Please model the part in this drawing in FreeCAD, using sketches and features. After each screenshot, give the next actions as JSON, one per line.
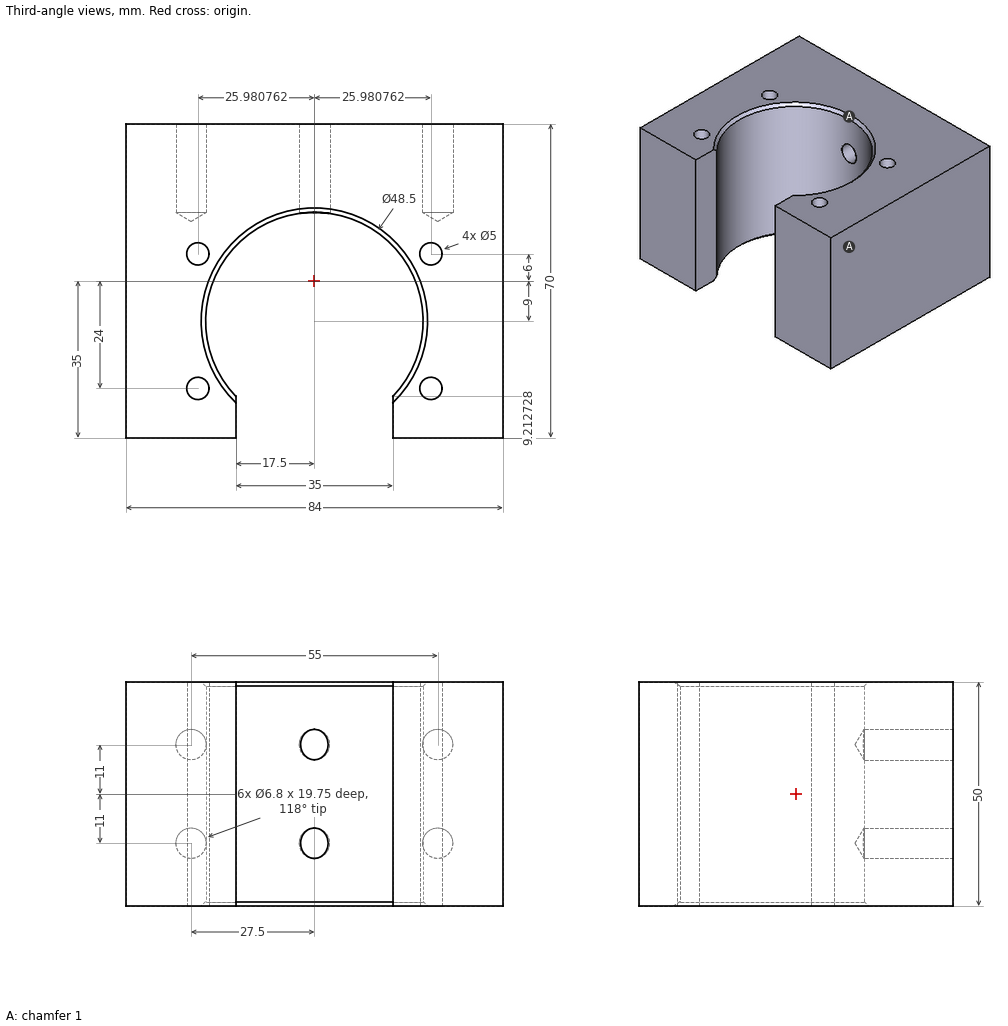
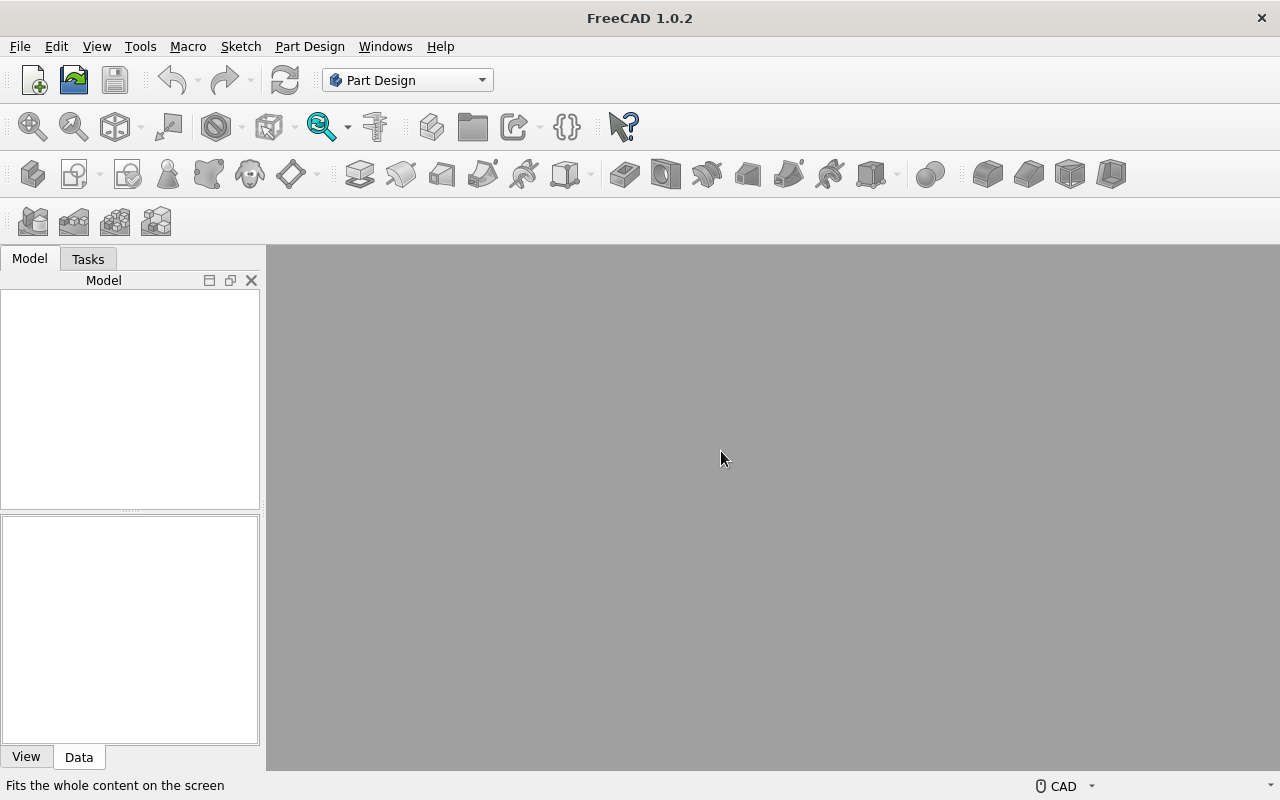
{"action": "left_click", "coordinate": [33, 80]}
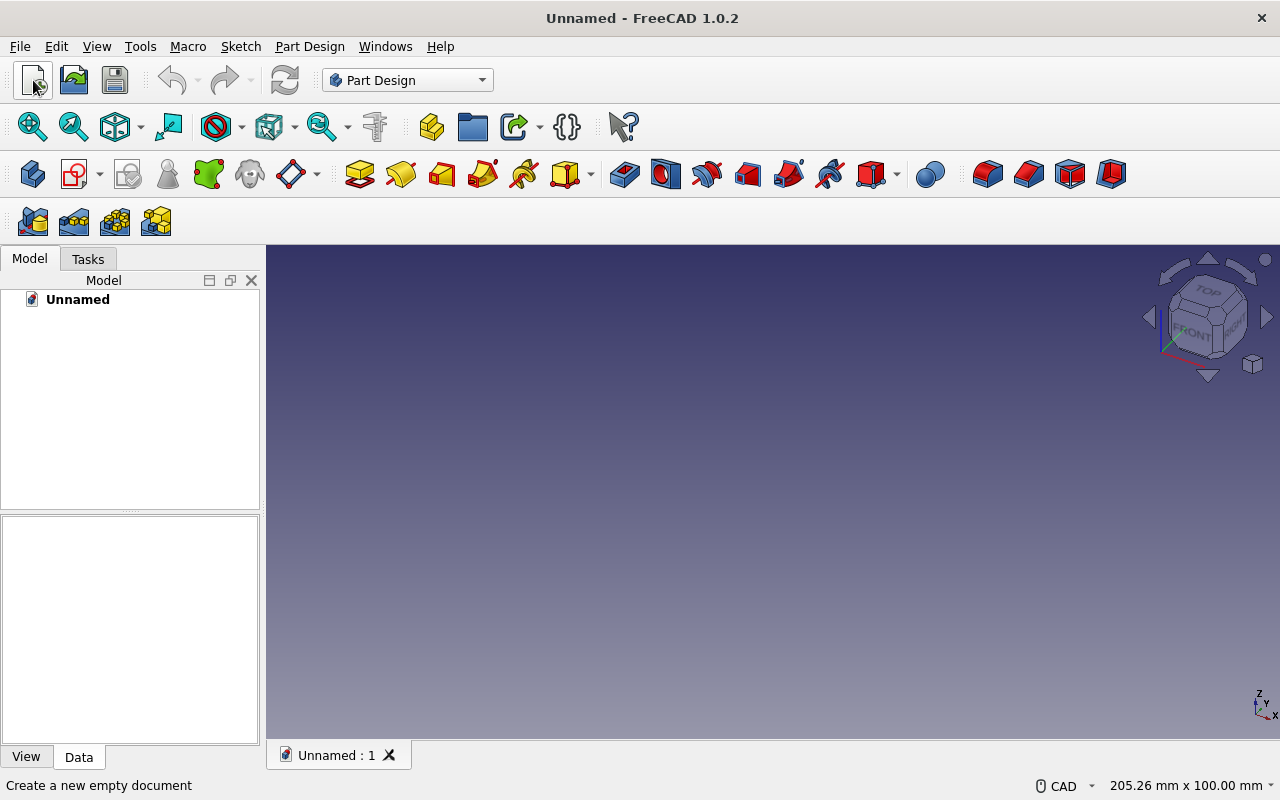
{"action": "left_click", "coordinate": [74, 174]}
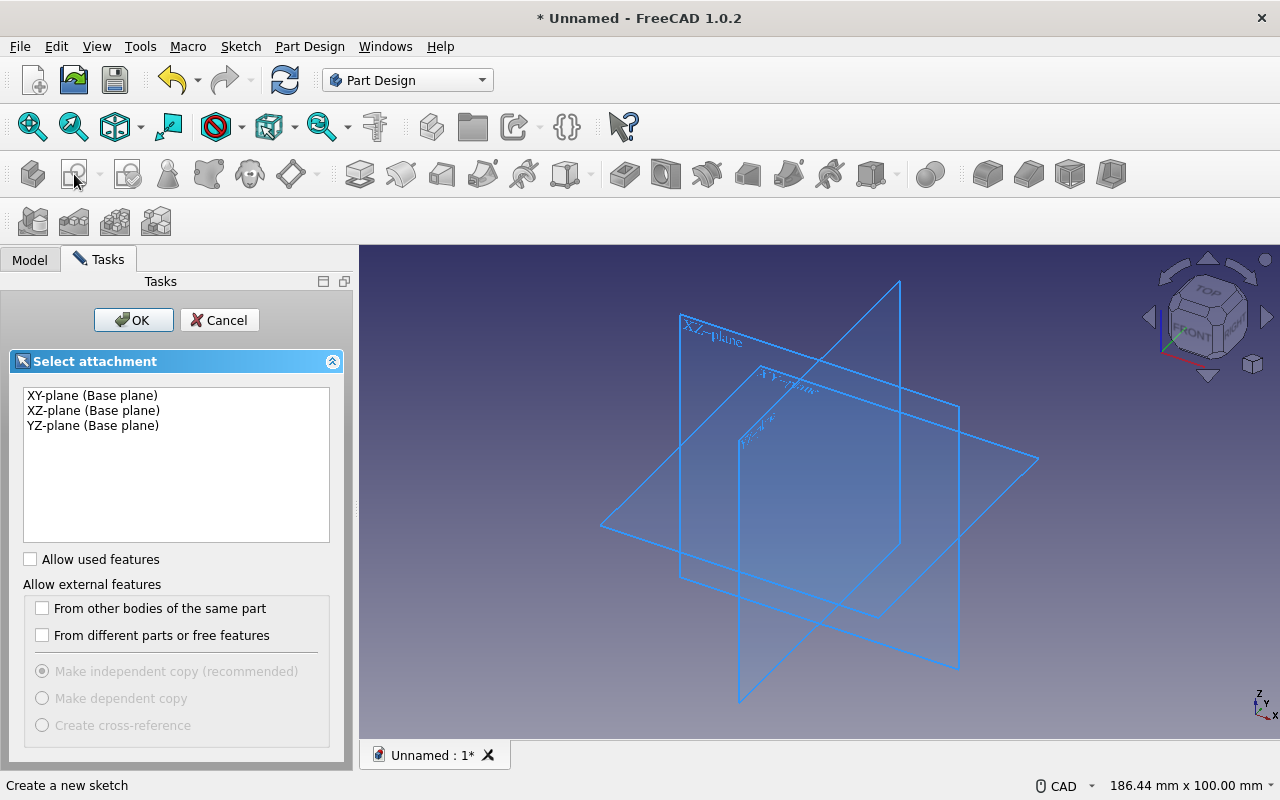
{"action": "left_click", "coordinate": [84, 396]}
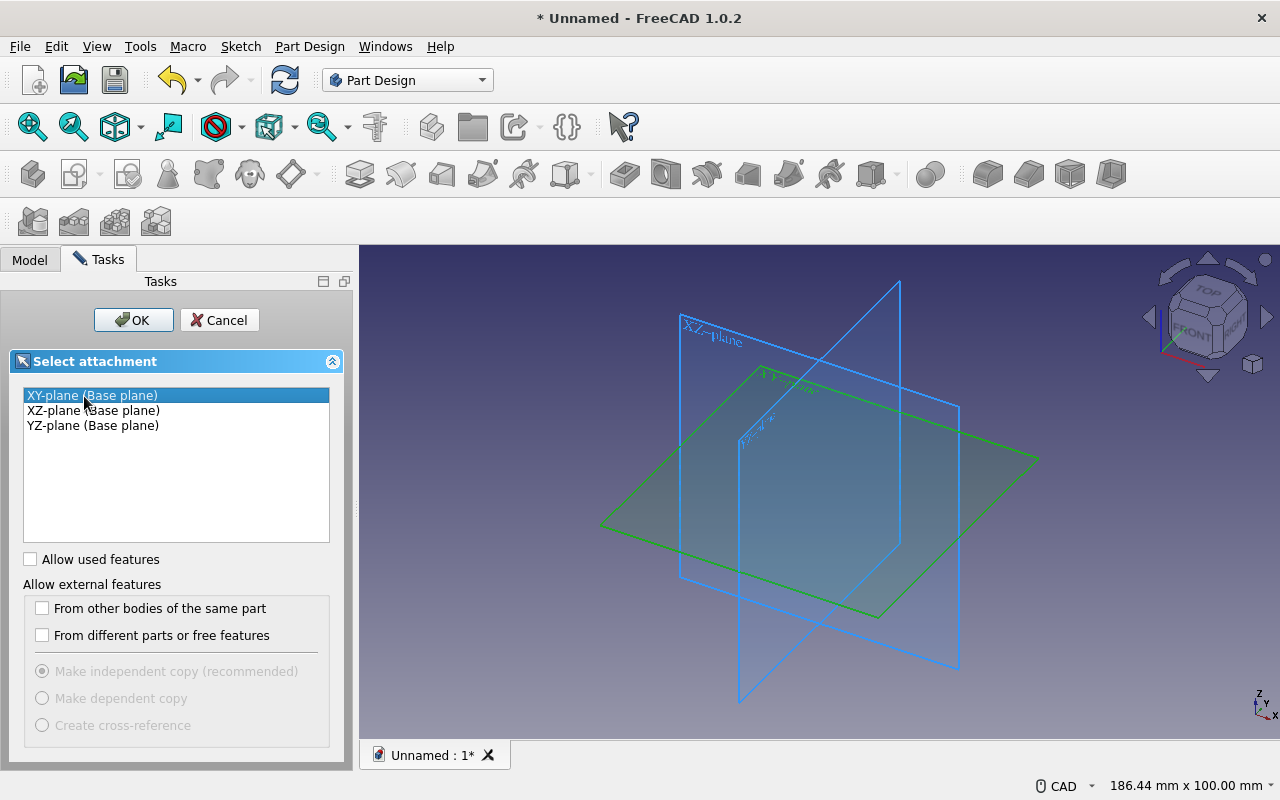
{"action": "left_click", "coordinate": [134, 320]}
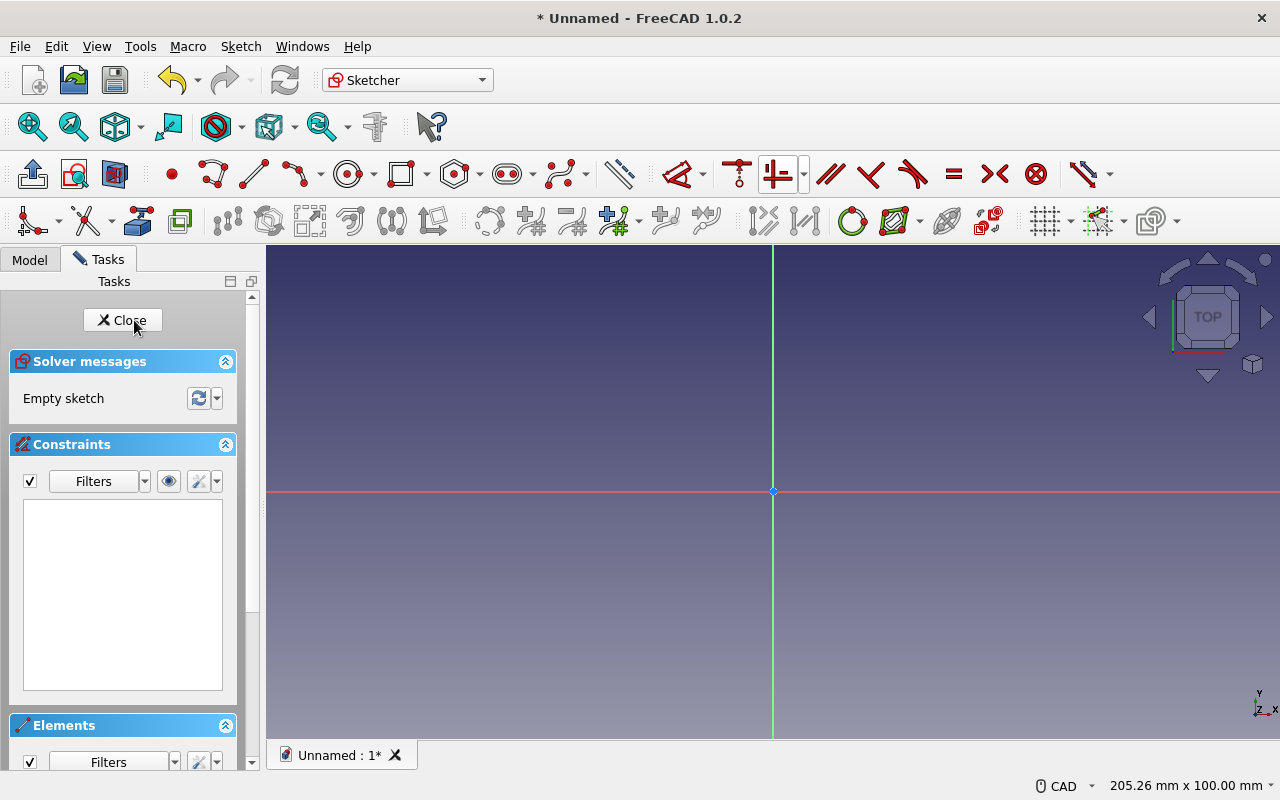
{"action": "left_click", "coordinate": [426, 174]}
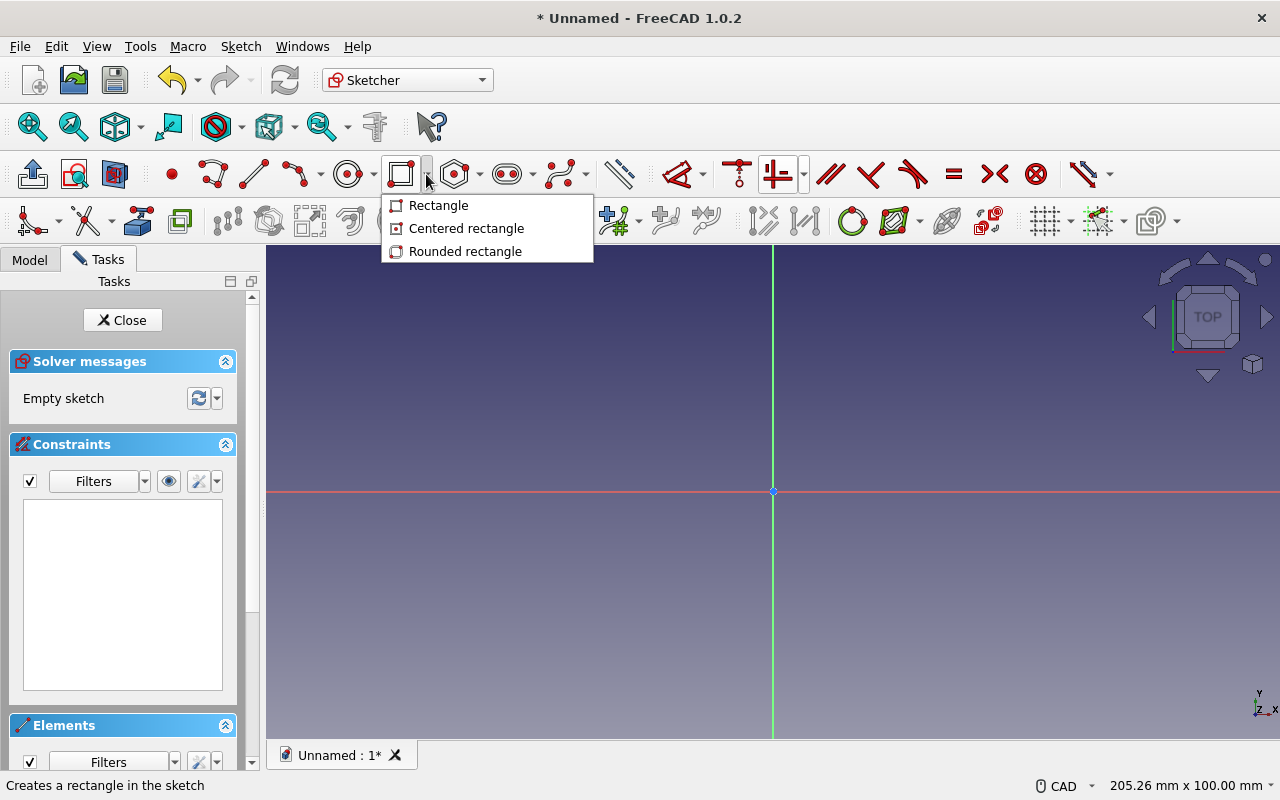
{"action": "left_click", "coordinate": [488, 228]}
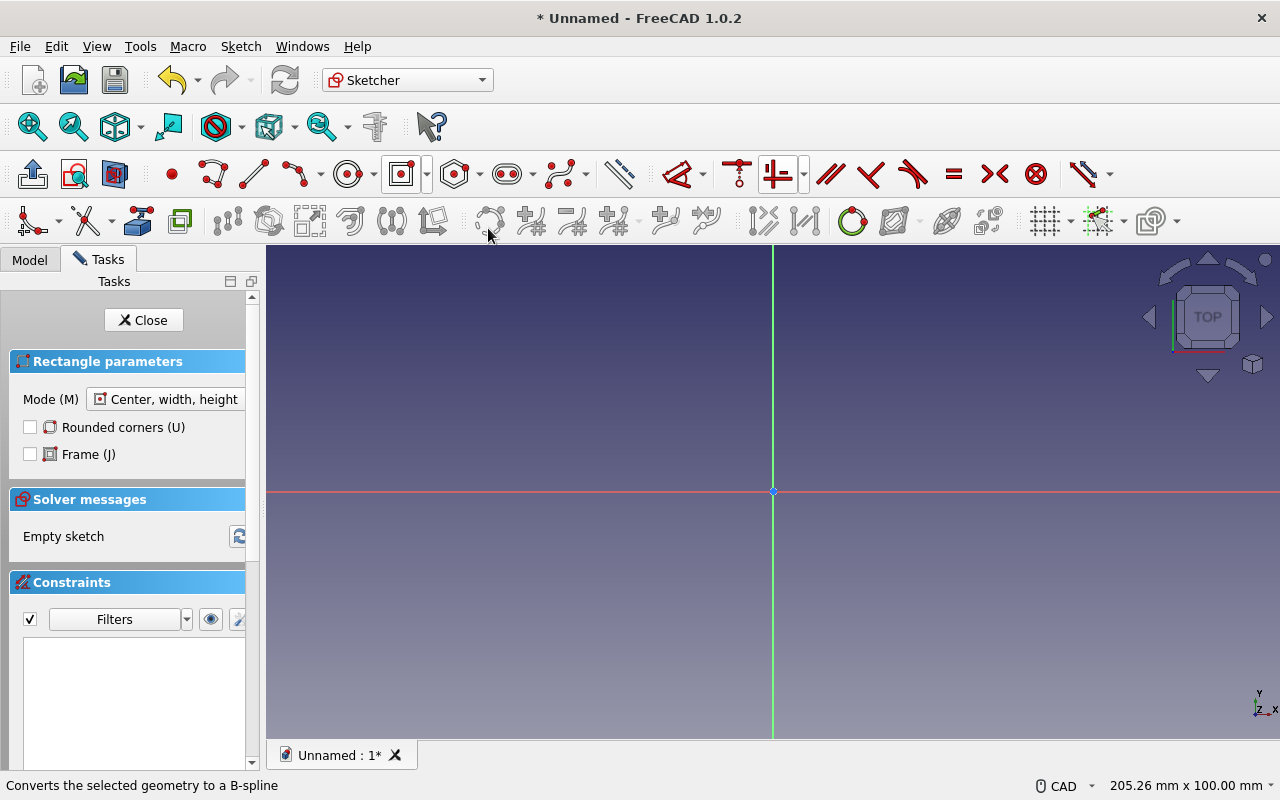
{"action": "left_click", "coordinate": [773, 492]}
{"action": "mouse_move", "coordinate": [980, 319]}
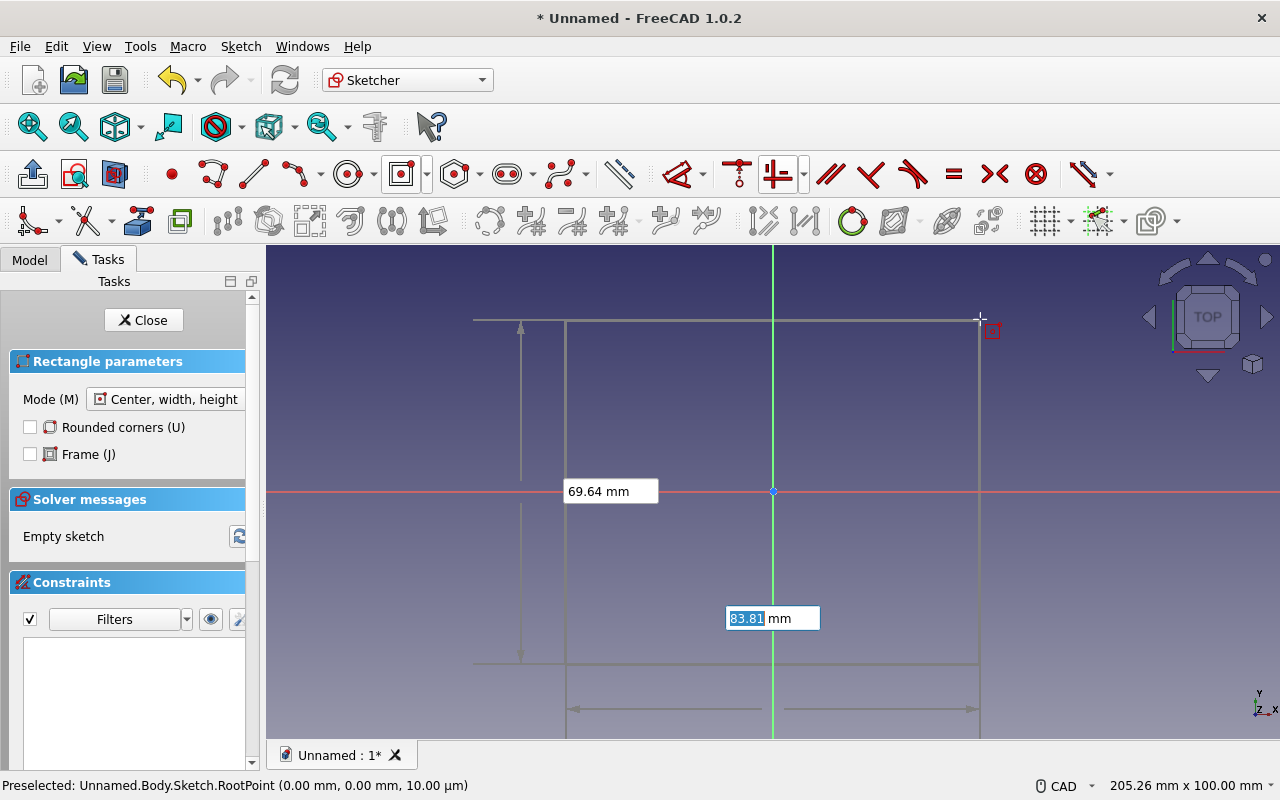
{"action": "type", "text": "84"}
{"action": "key", "text": "Tab"}
{"action": "type", "text": "70"}
{"action": "key", "text": "Return"}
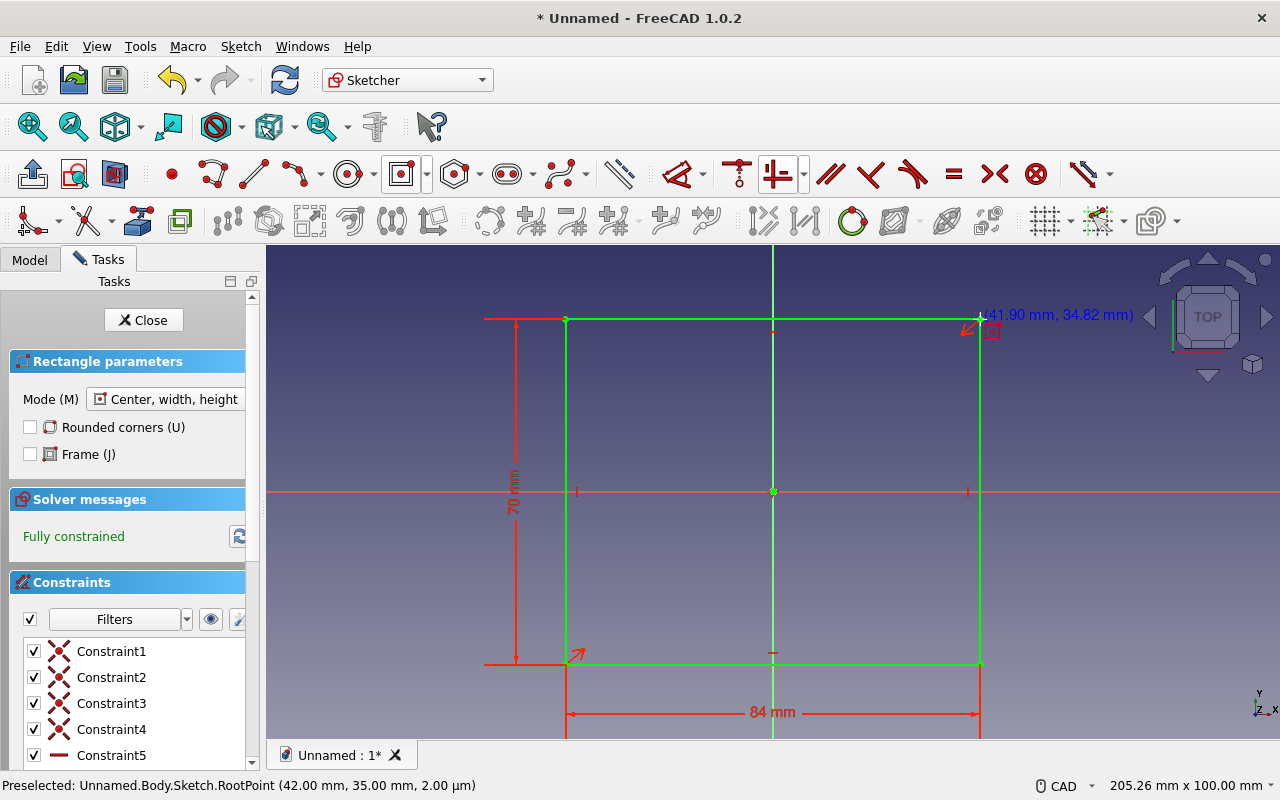
{"action": "key", "text": "g c"}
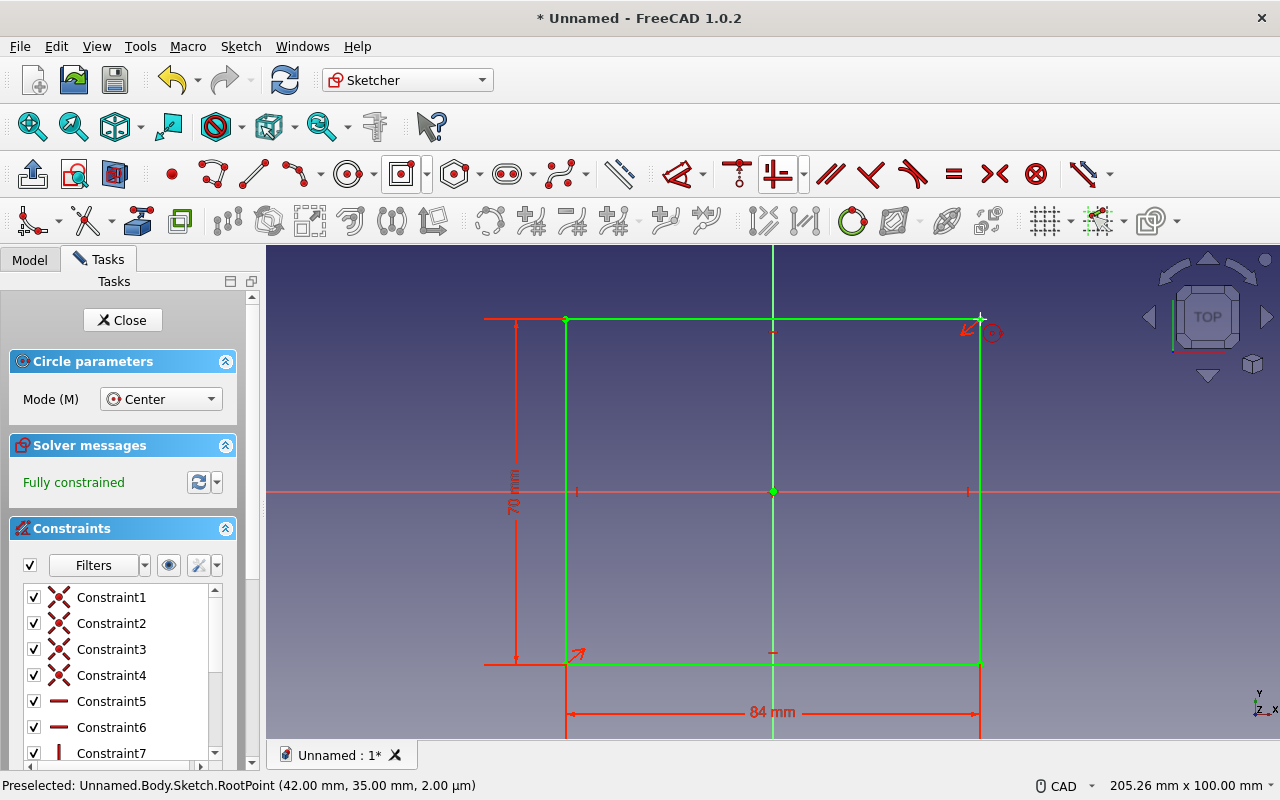
{"action": "left_click", "coordinate": [773, 536]}
{"action": "mouse_move", "coordinate": [858, 452]}